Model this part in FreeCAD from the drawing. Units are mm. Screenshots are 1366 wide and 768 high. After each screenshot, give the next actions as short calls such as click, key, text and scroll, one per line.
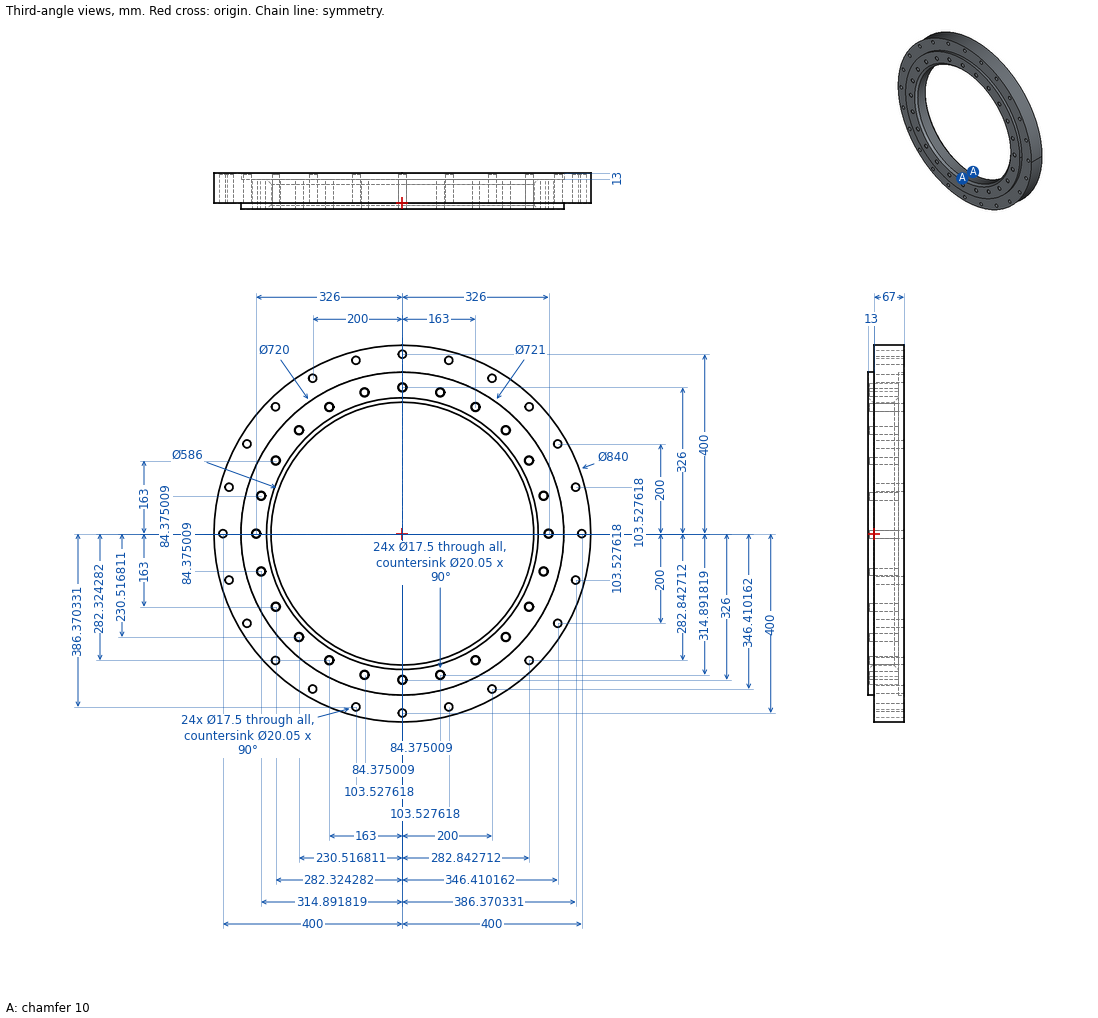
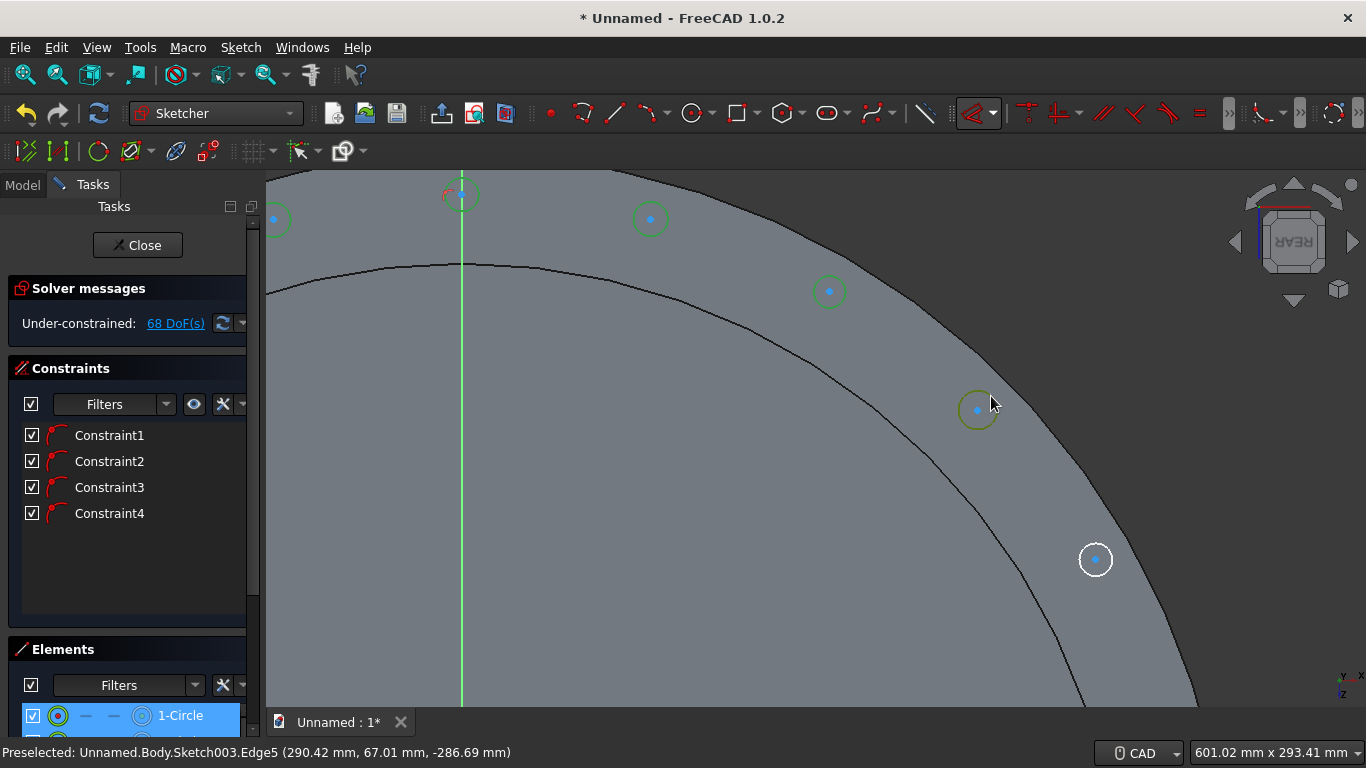
click(1107, 548)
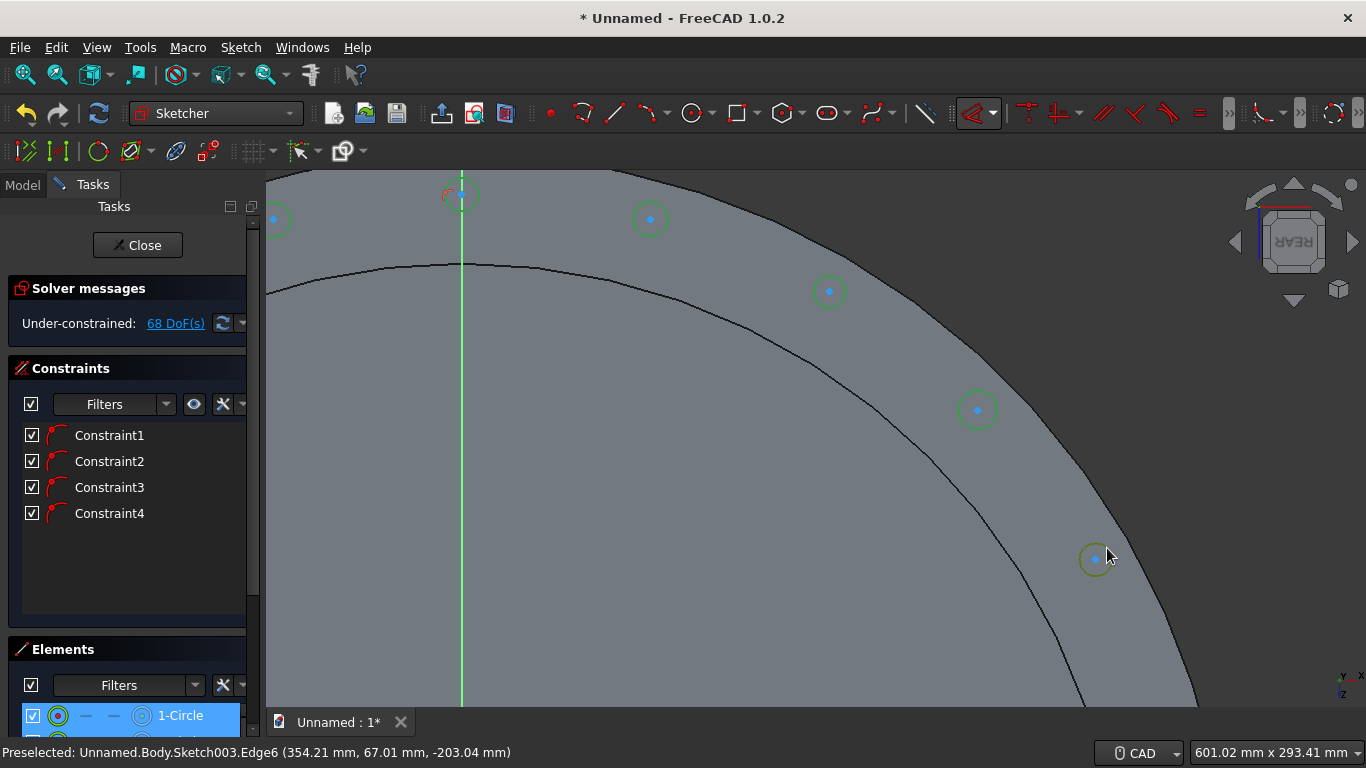
scroll(841, 280, down, 7)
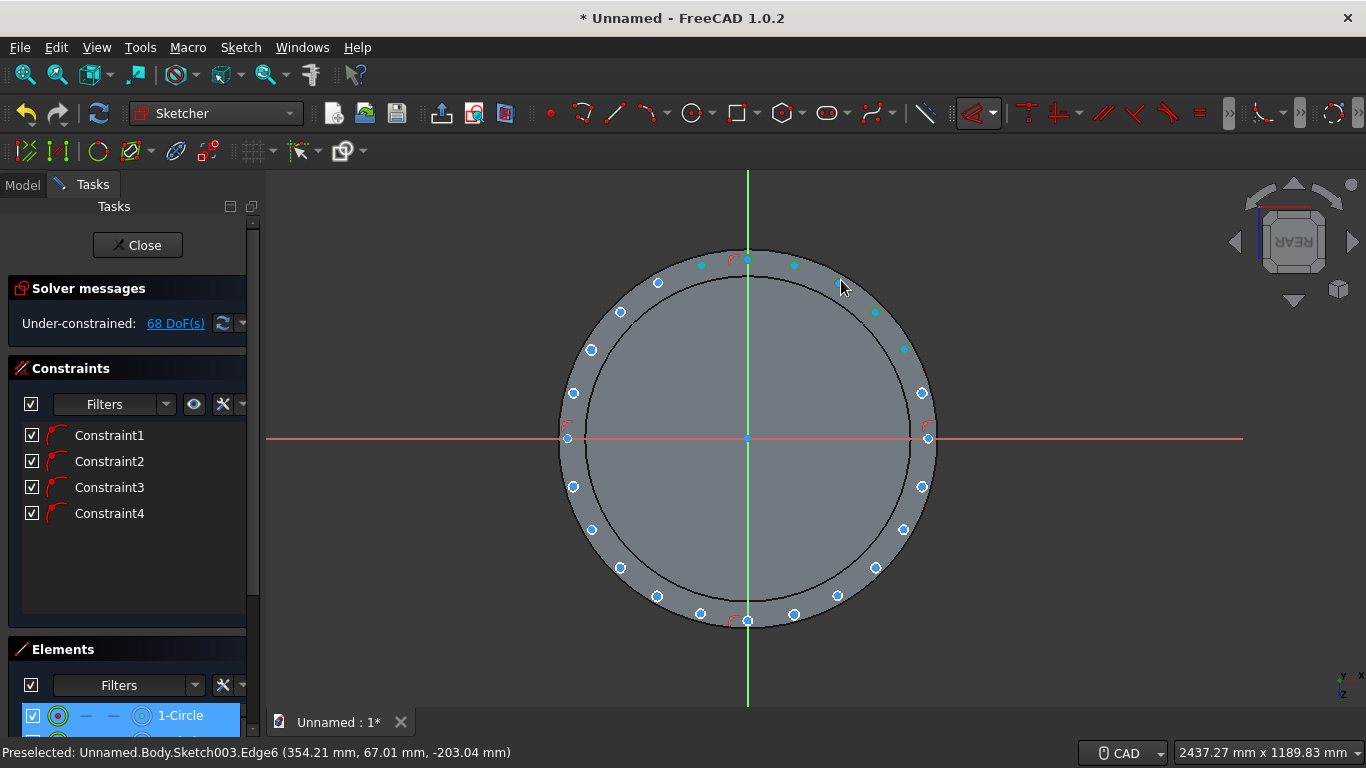
scroll(925, 390, up, 6)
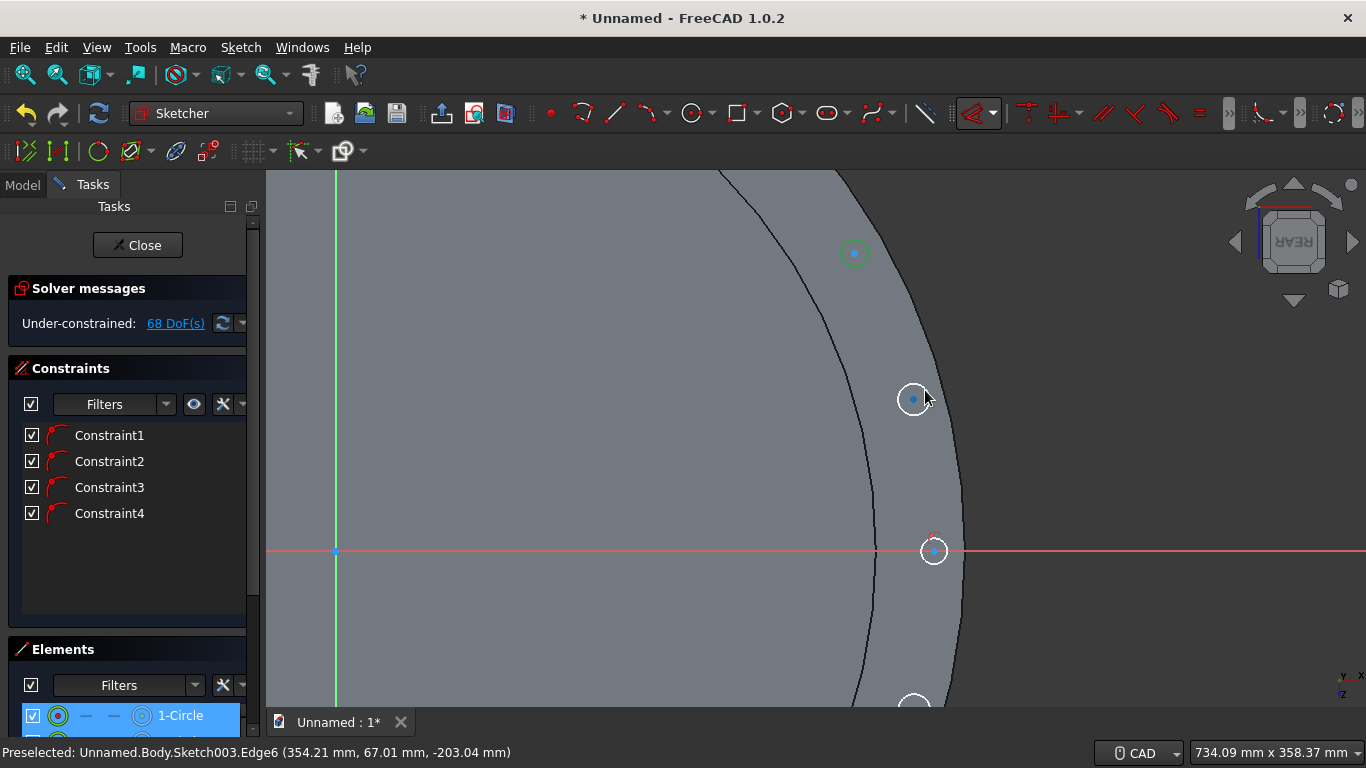
click(925, 388)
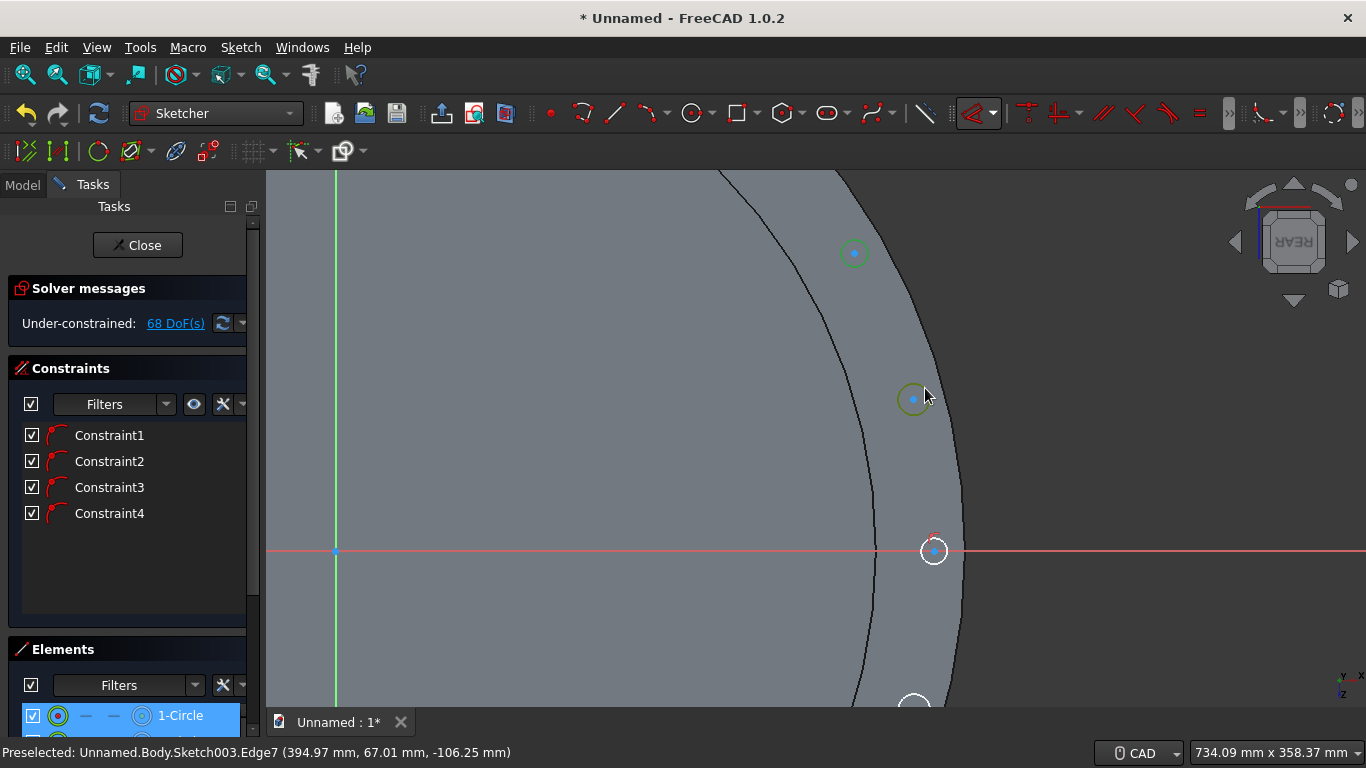
scroll(943, 542, up, 3)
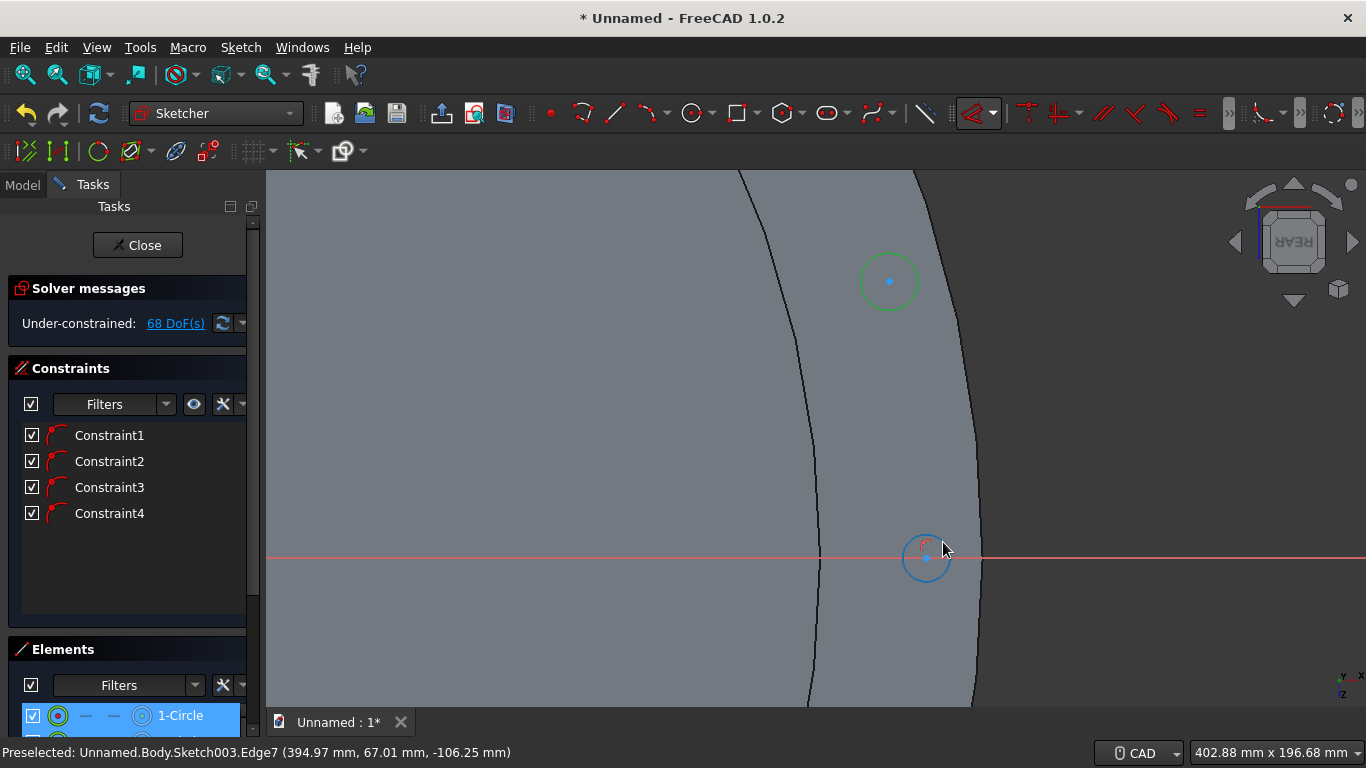
click(943, 542)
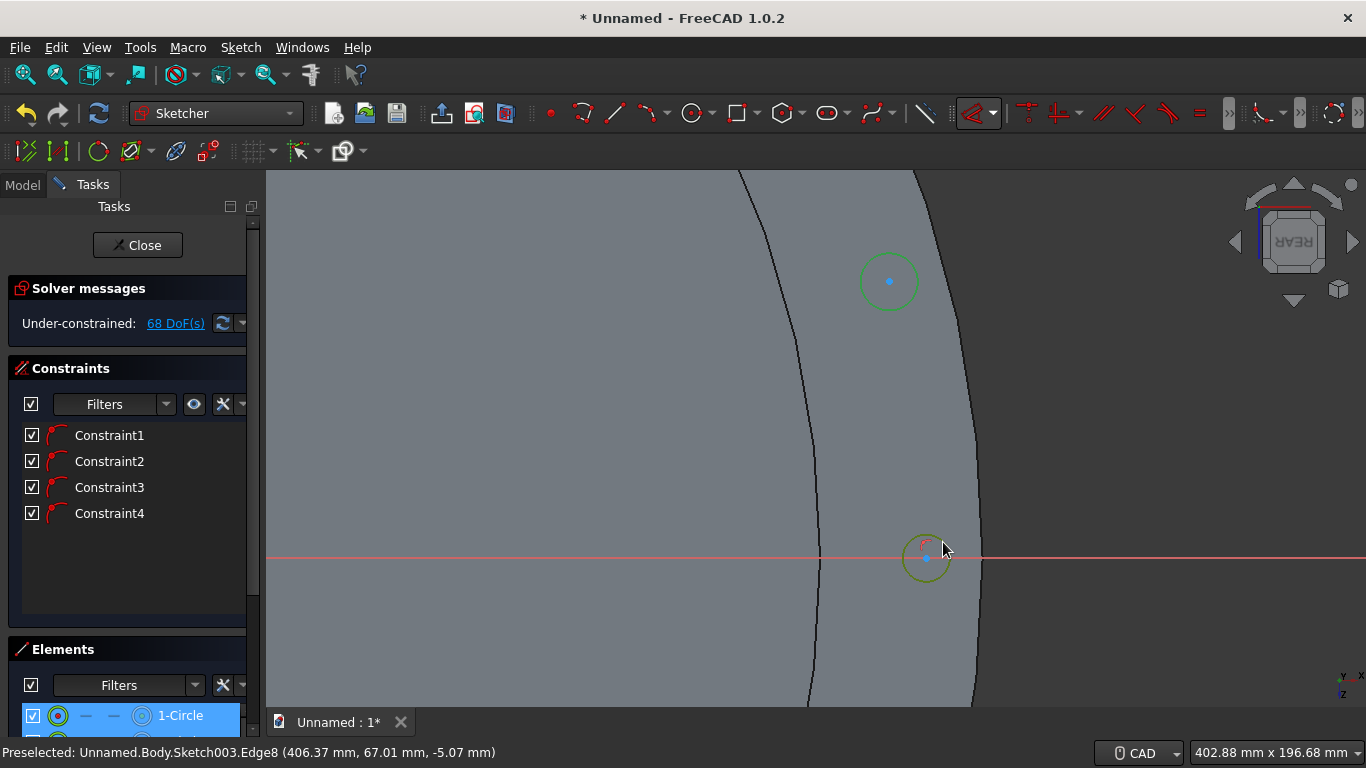
scroll(928, 415, down, 9)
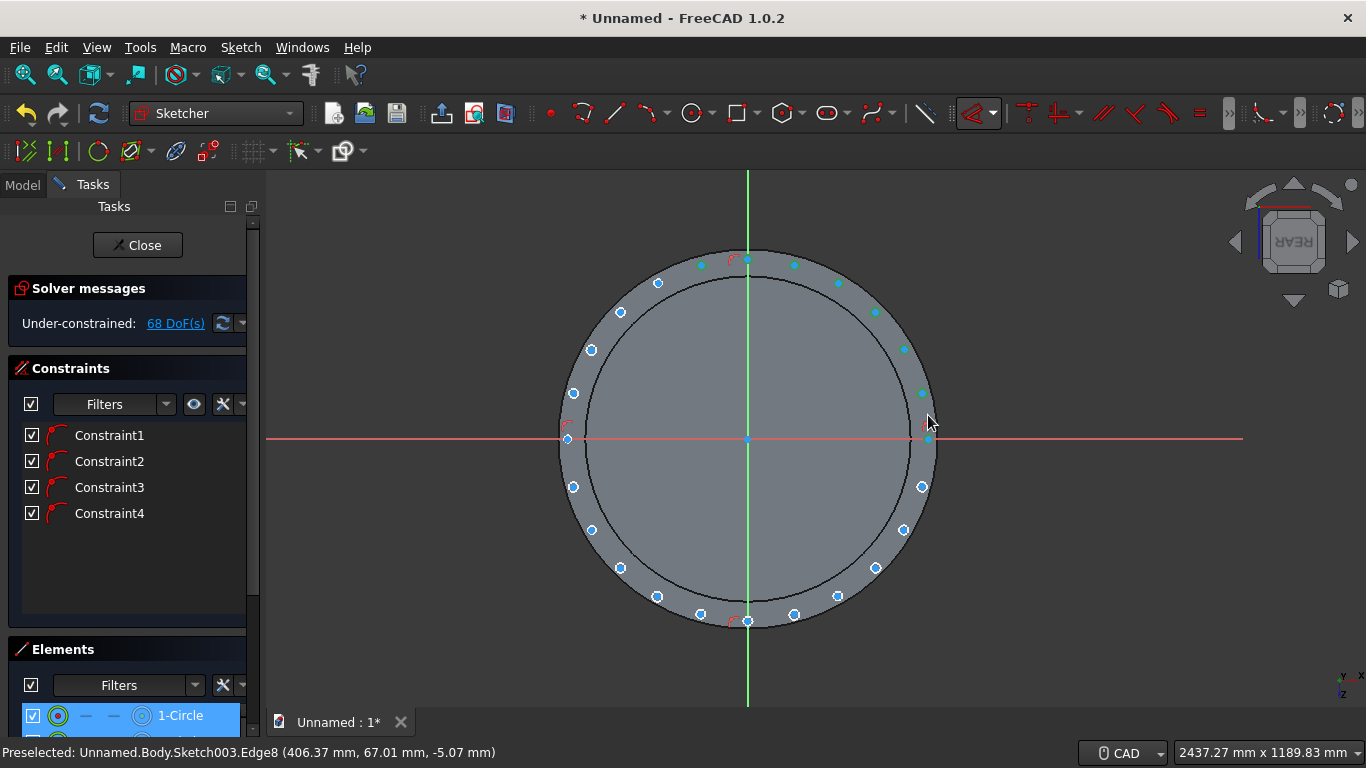
scroll(926, 484, up, 6)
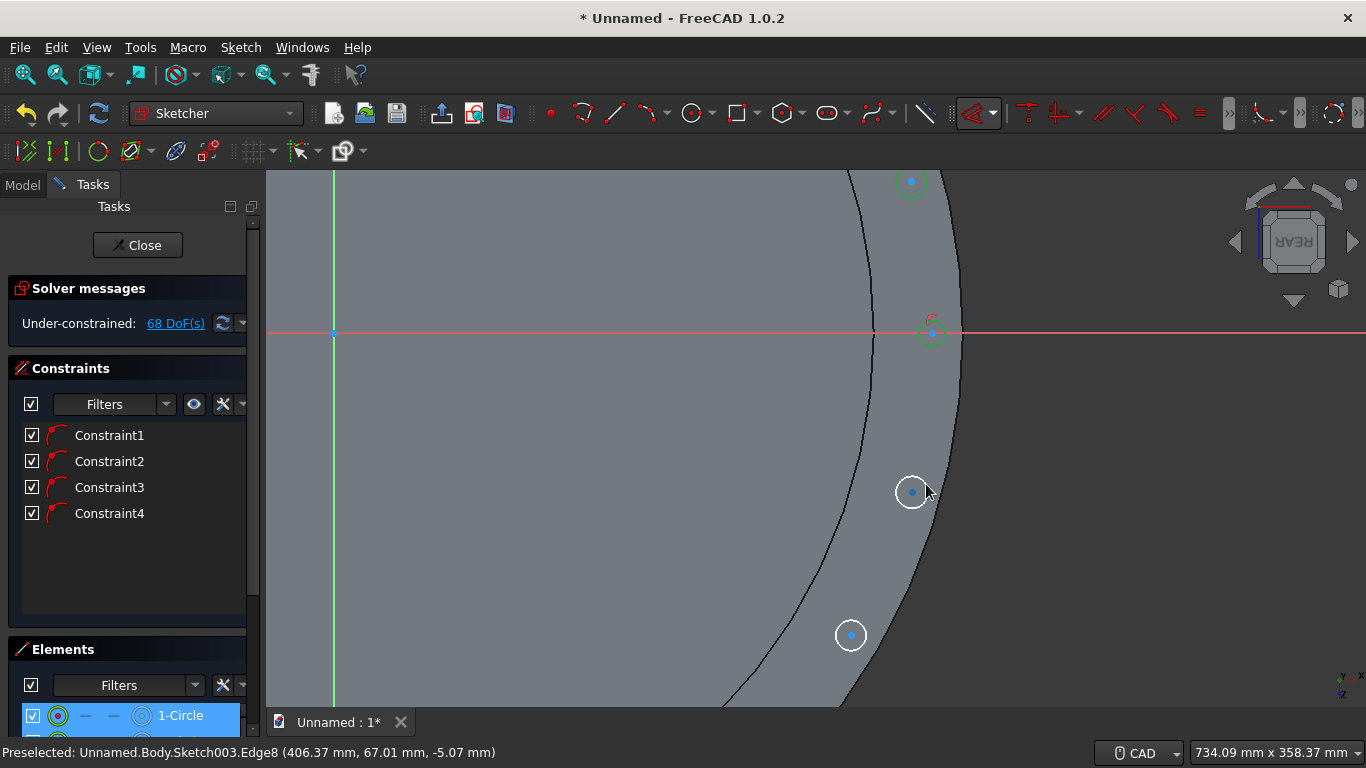
click(923, 481)